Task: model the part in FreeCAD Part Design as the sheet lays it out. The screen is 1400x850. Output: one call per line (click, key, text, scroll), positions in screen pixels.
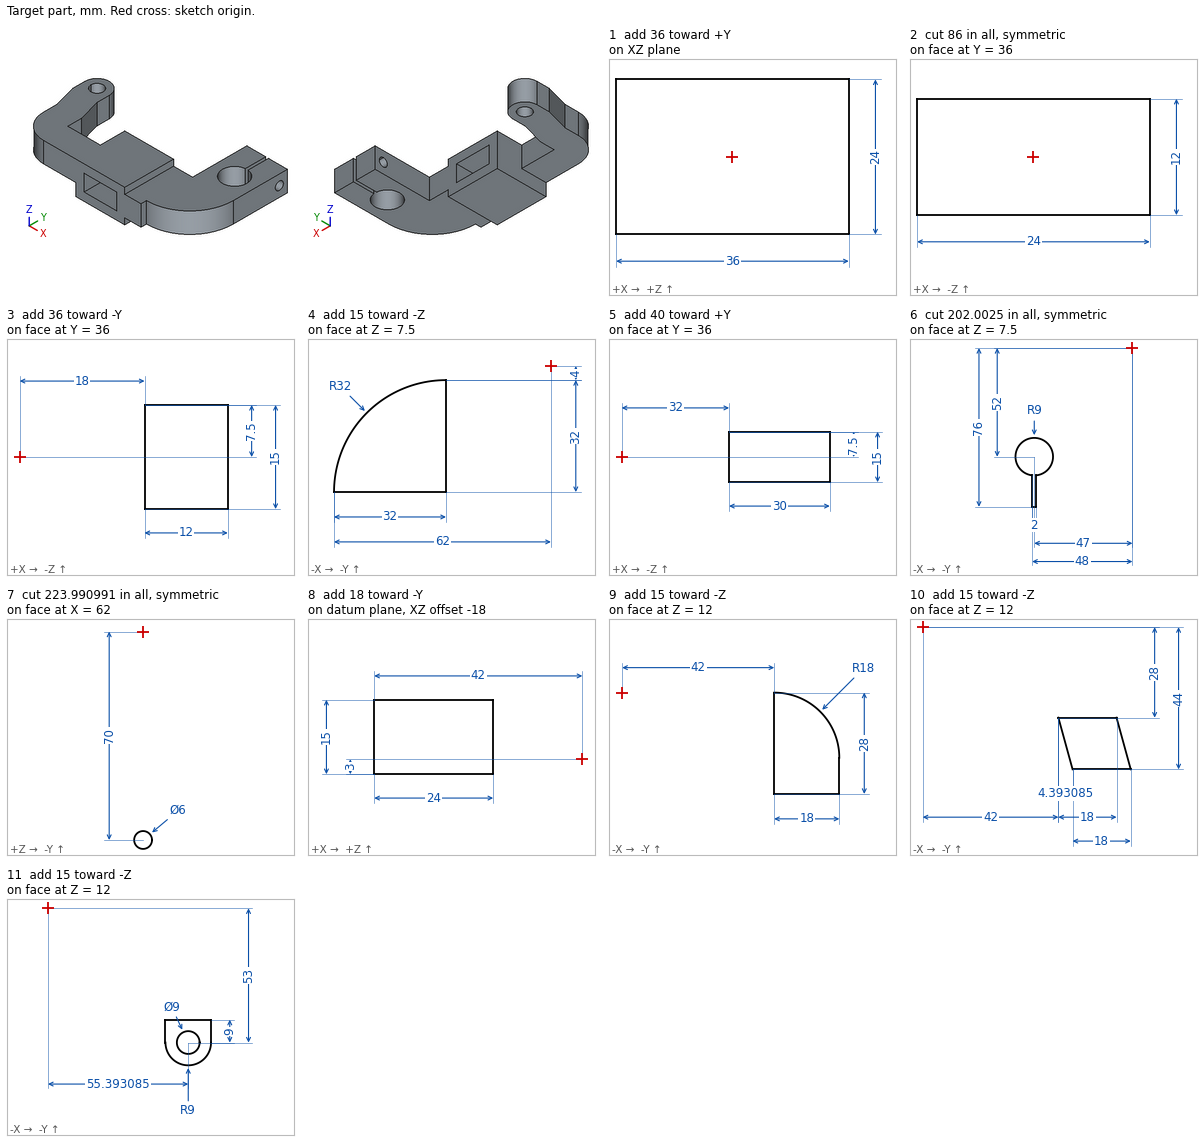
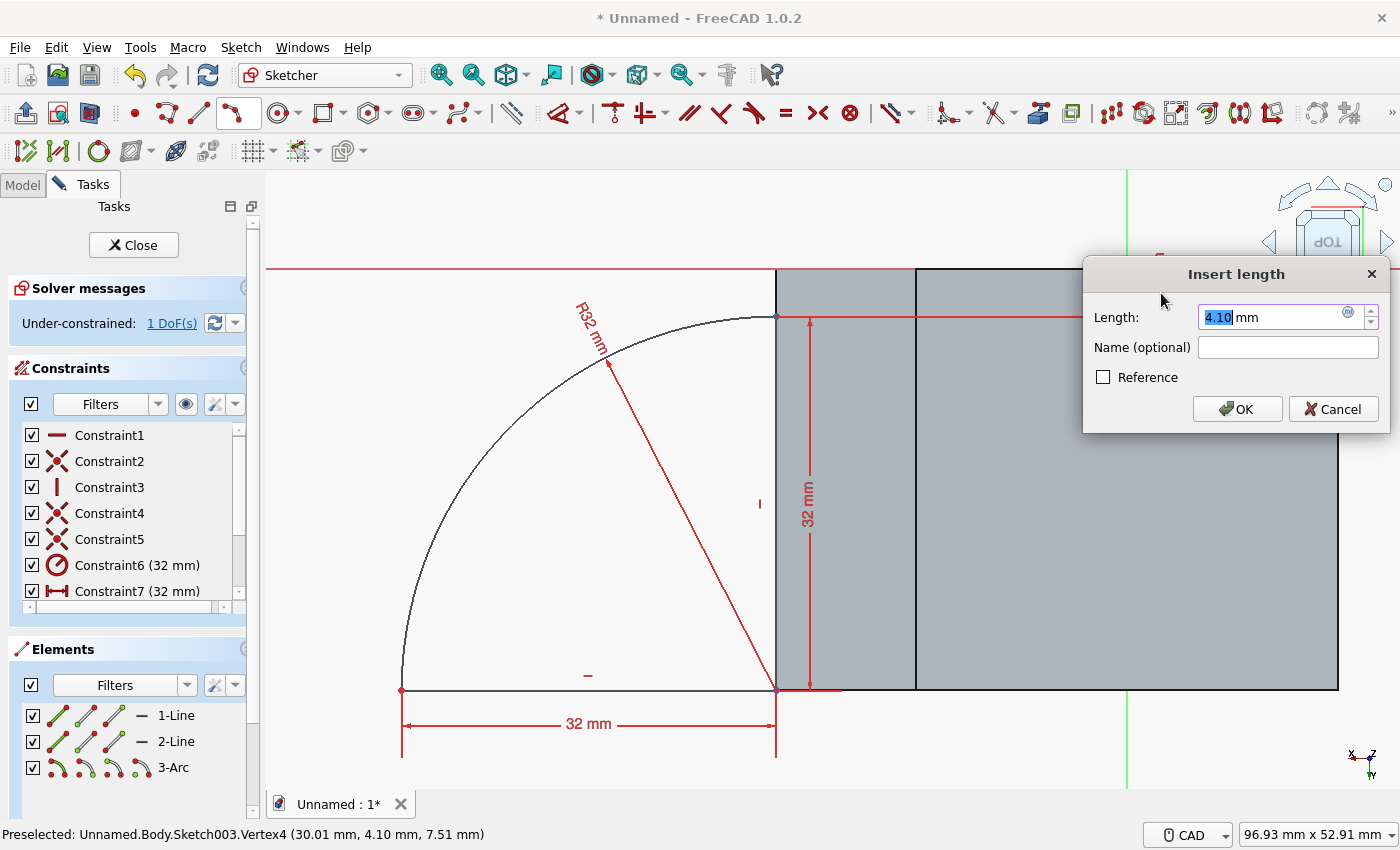
text(4)
key(Return)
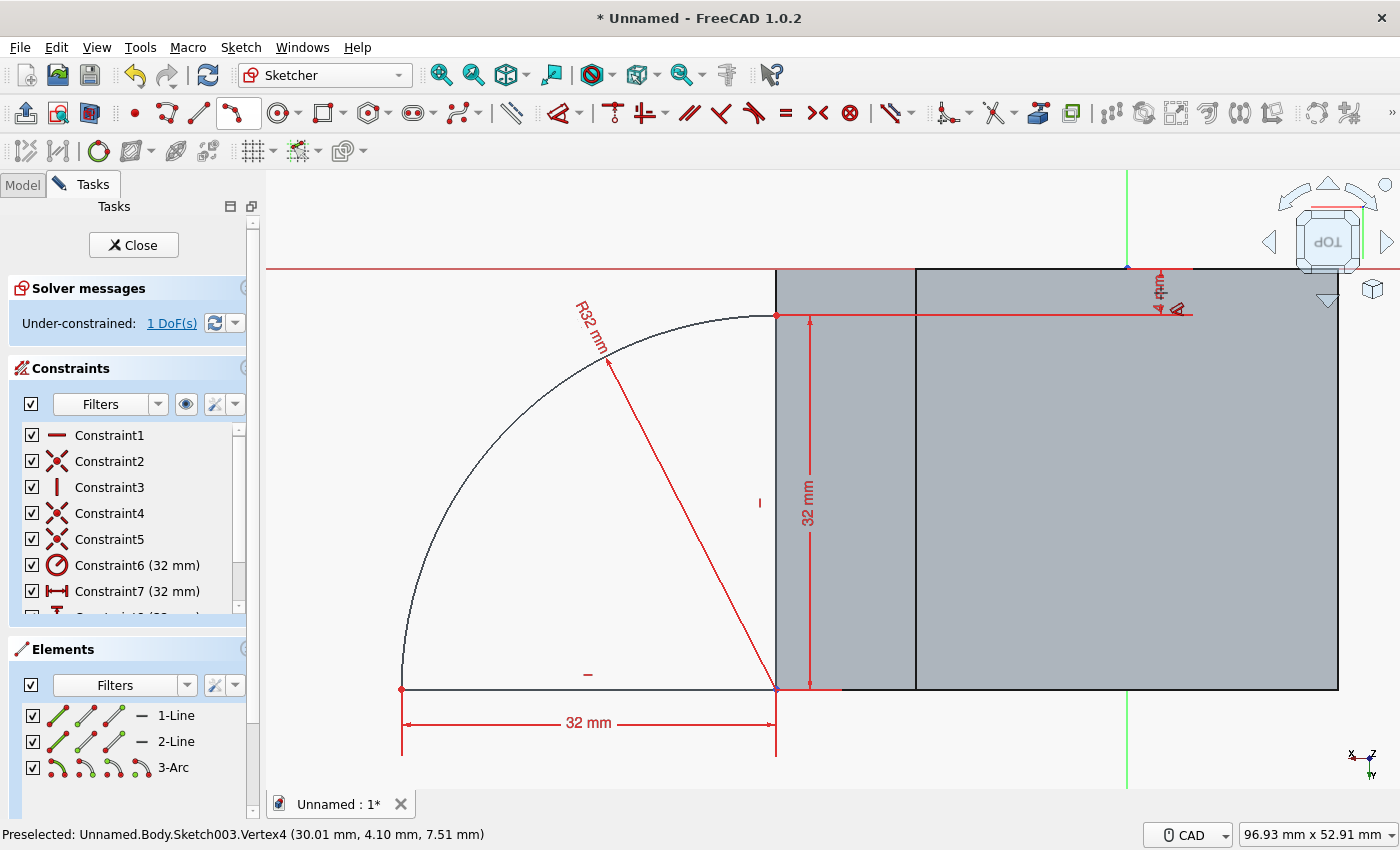
click(402, 690)
click(764, 724)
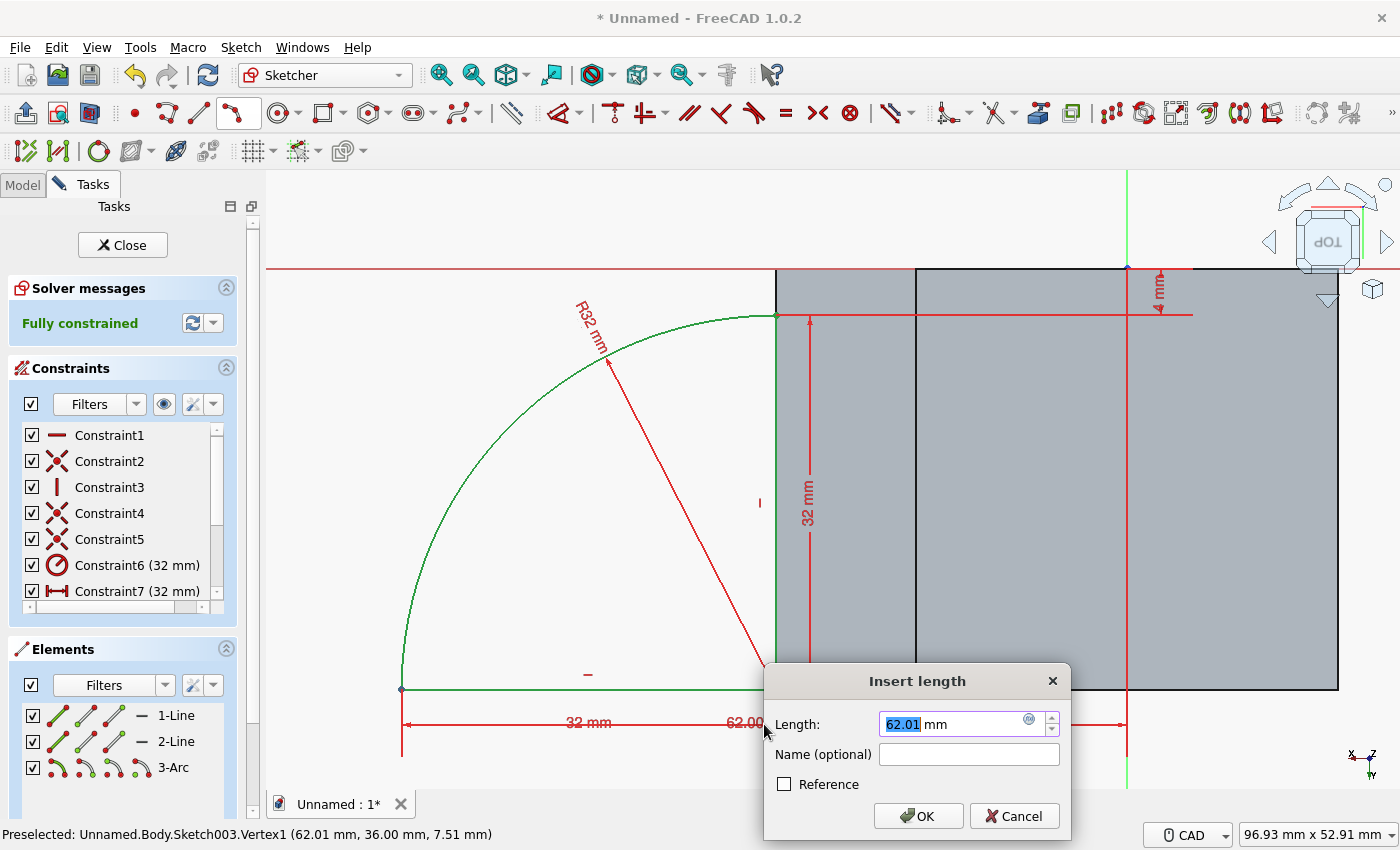
text(62)
key(Return)
key(Escape)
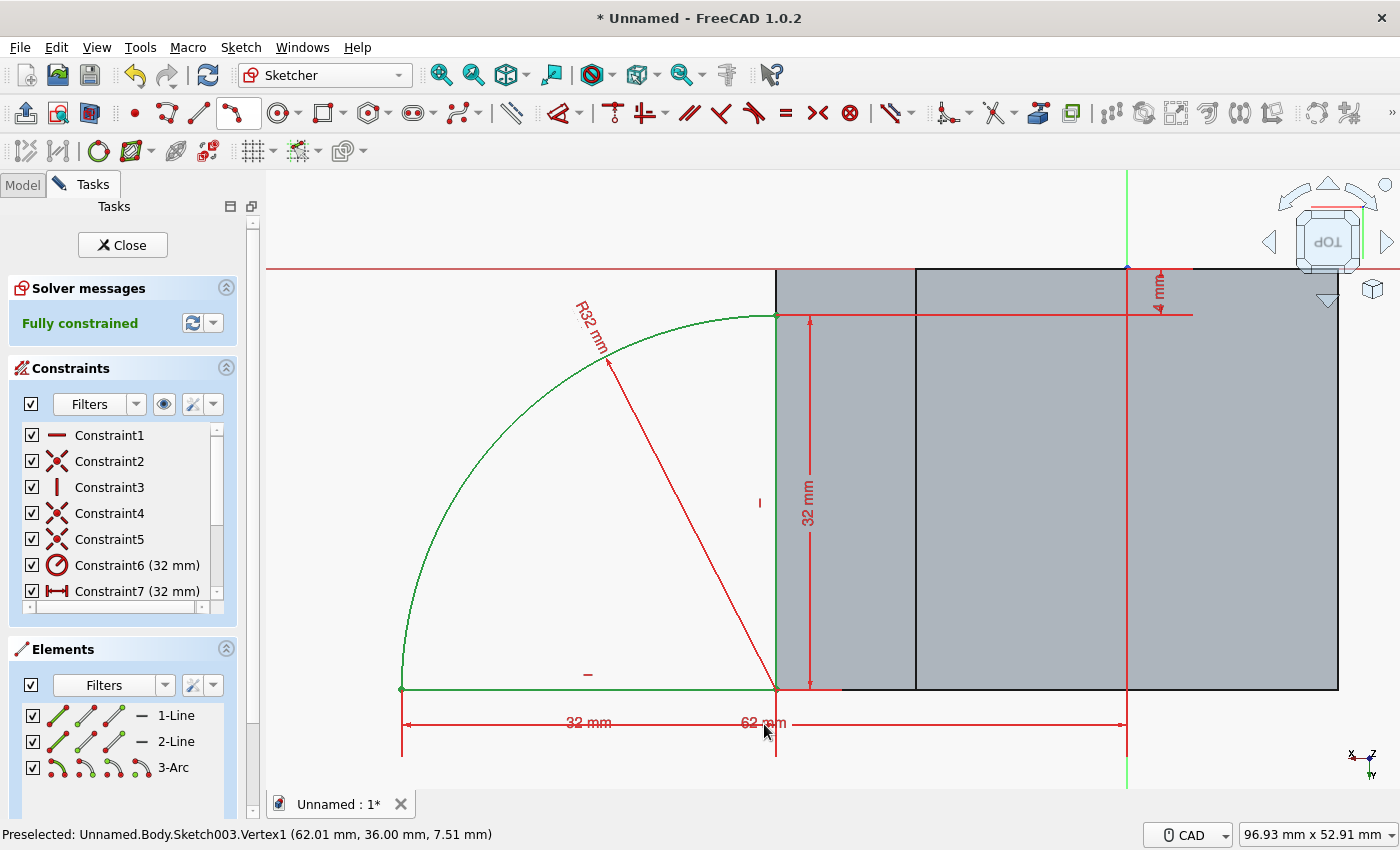
click(123, 245)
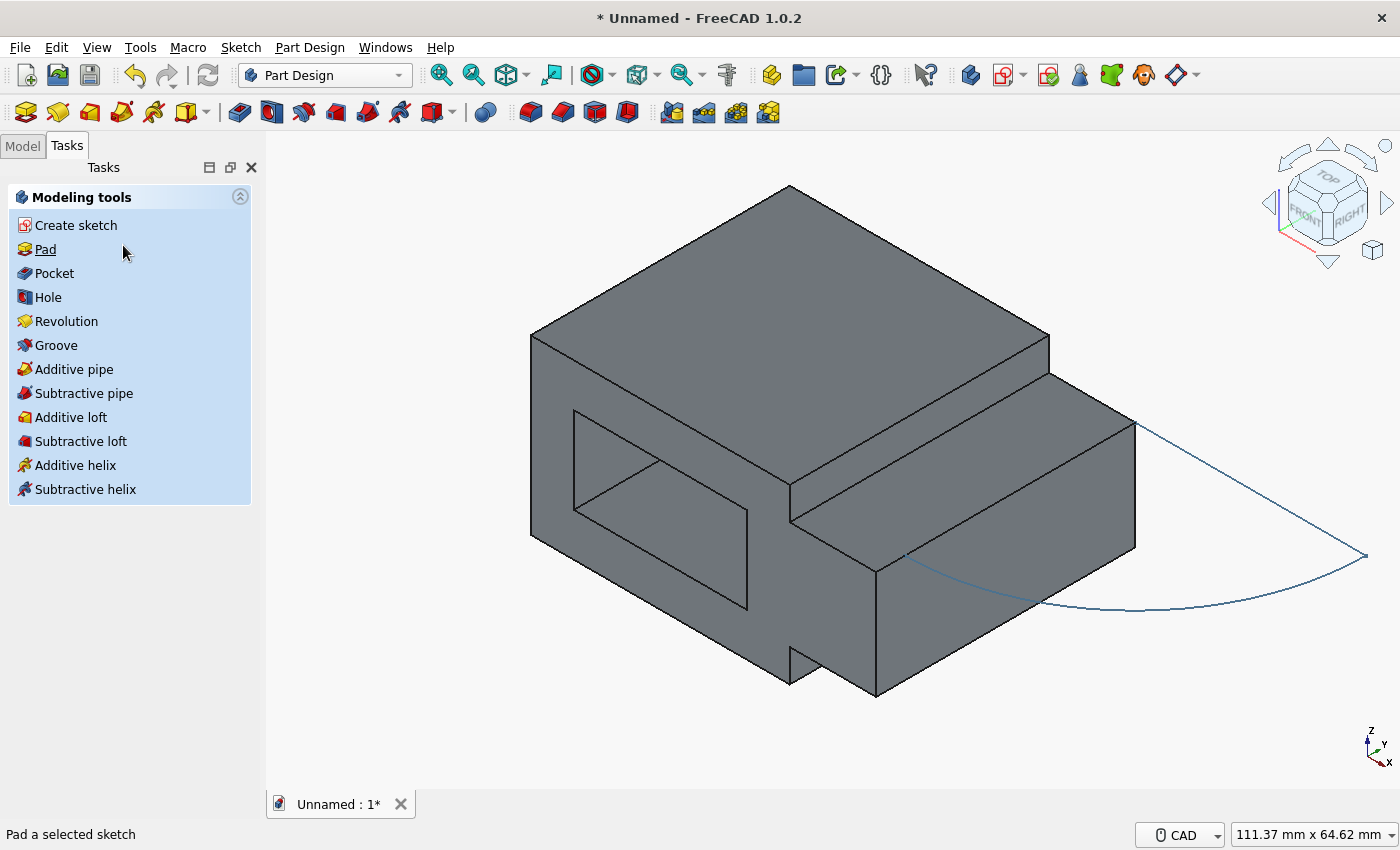
click(26, 112)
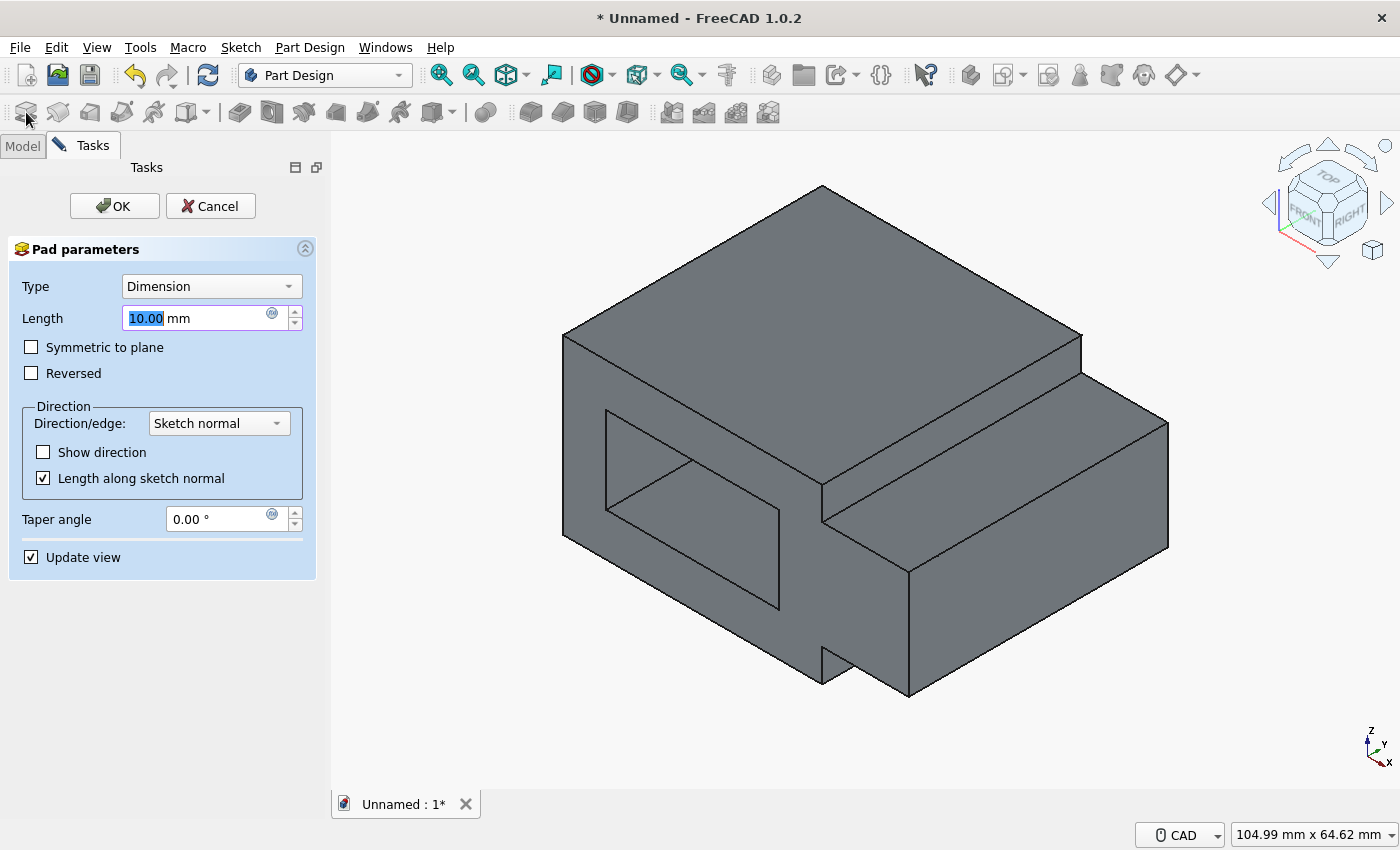
text(15)
key(Tab)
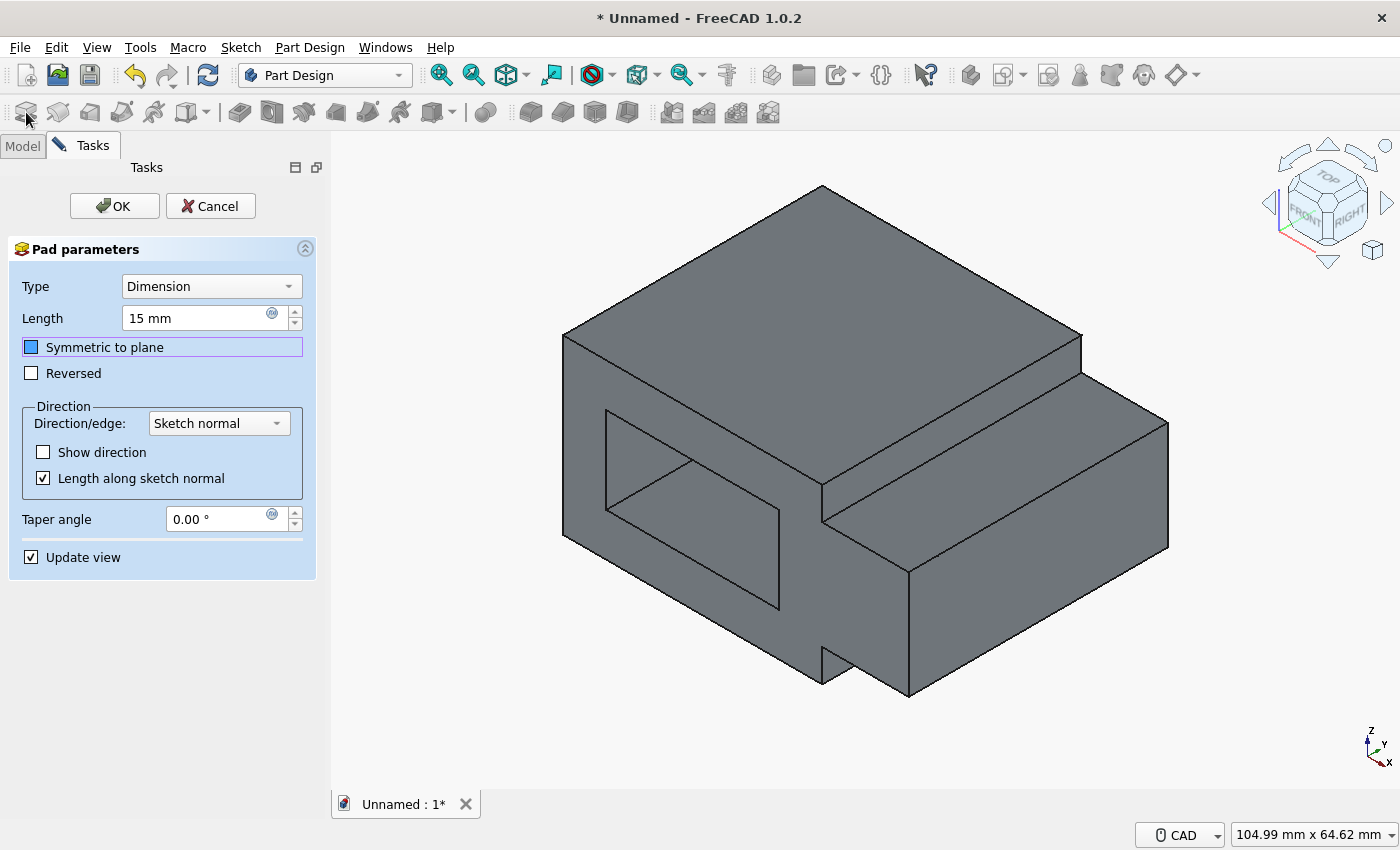
click(30, 373)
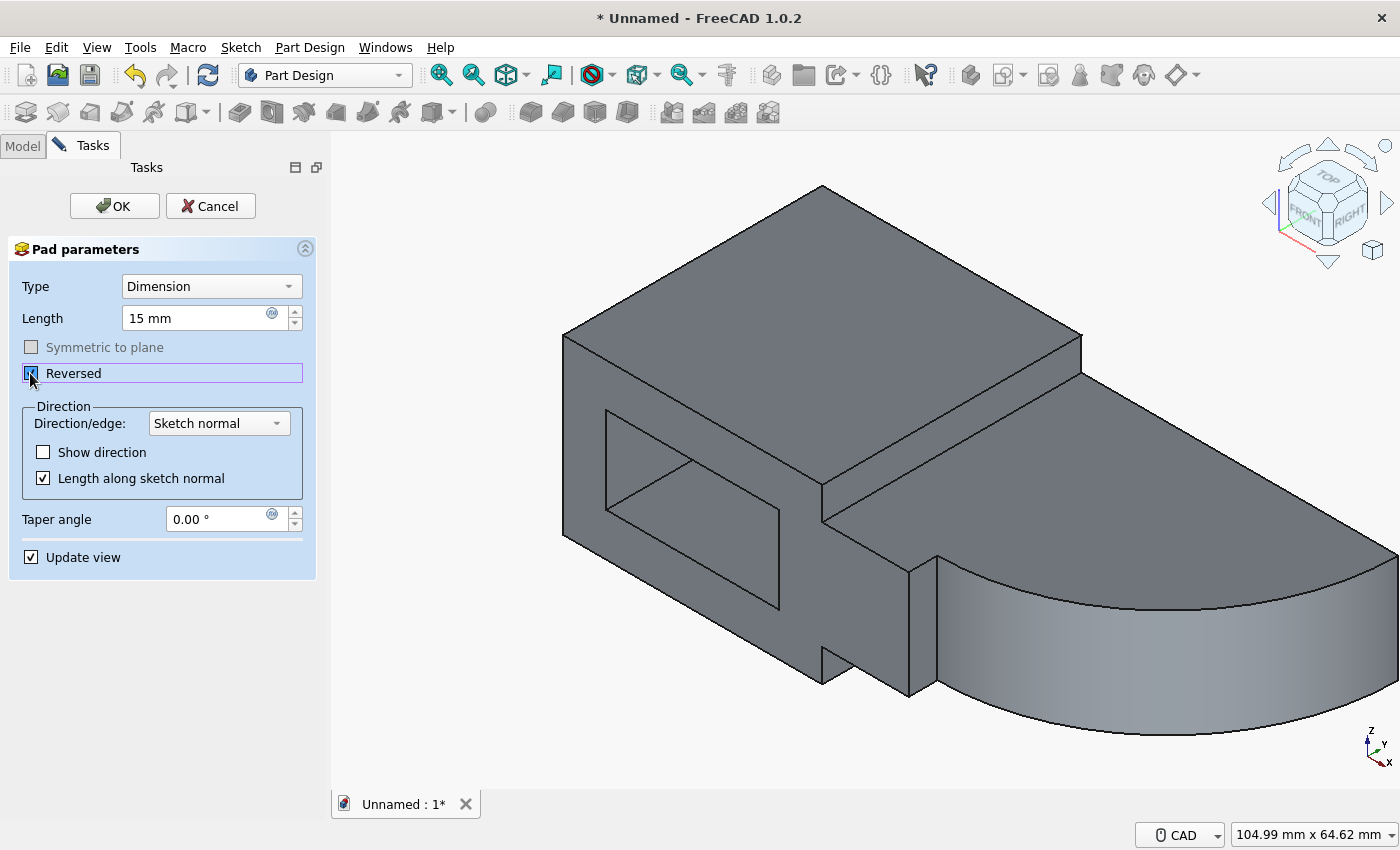
click(115, 206)